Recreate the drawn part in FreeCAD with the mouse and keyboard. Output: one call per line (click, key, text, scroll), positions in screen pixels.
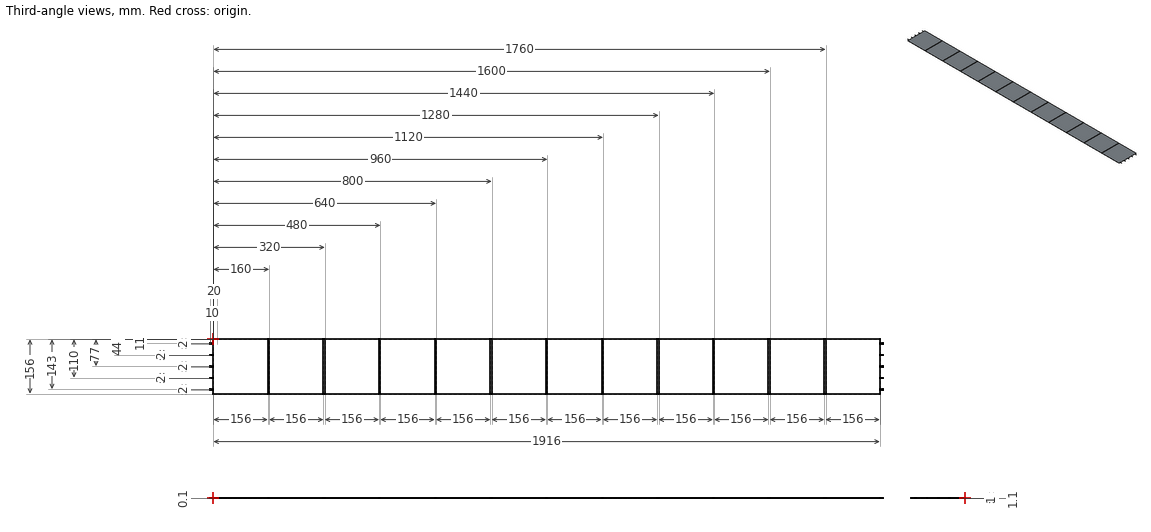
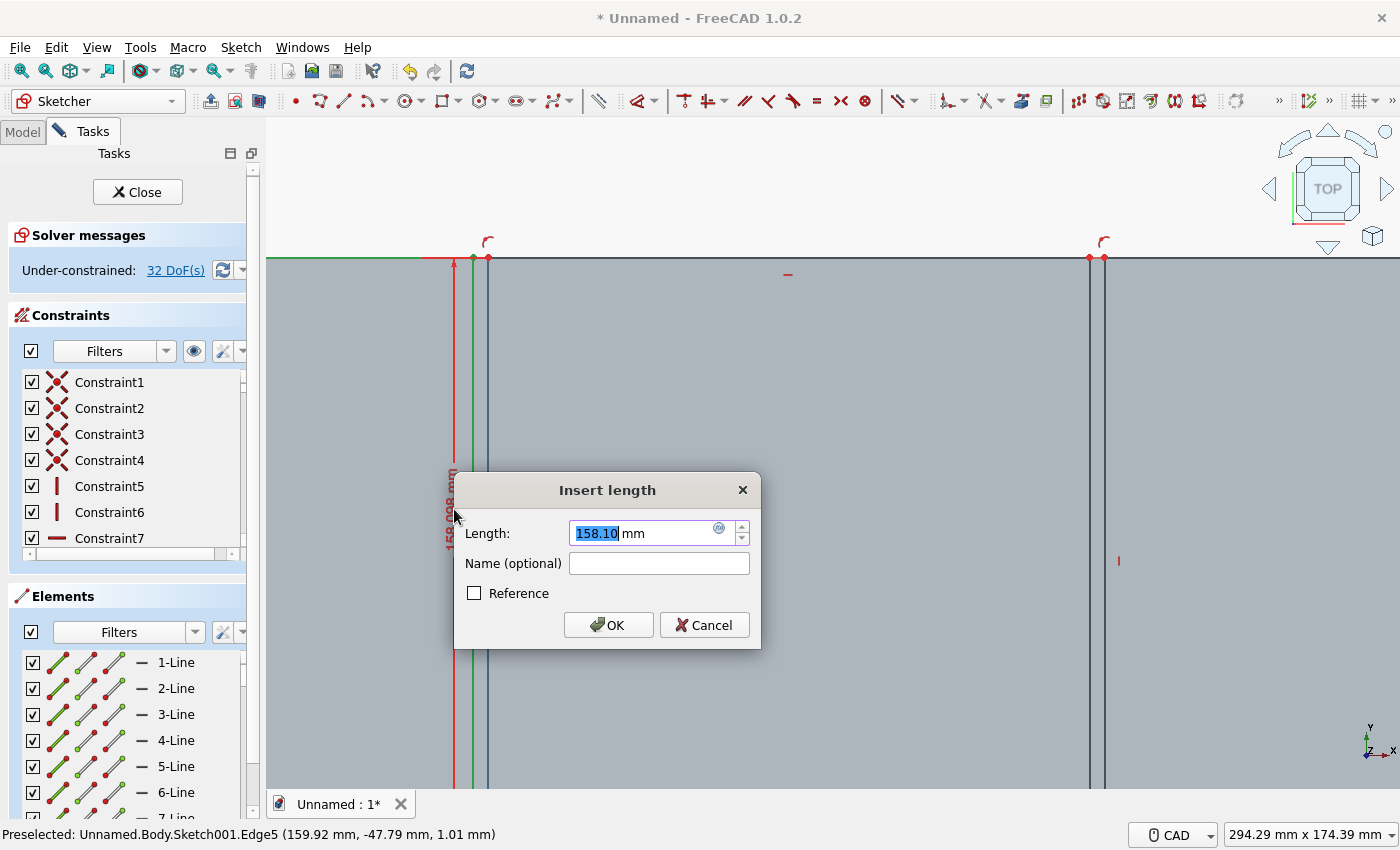
text(156)
key(Return)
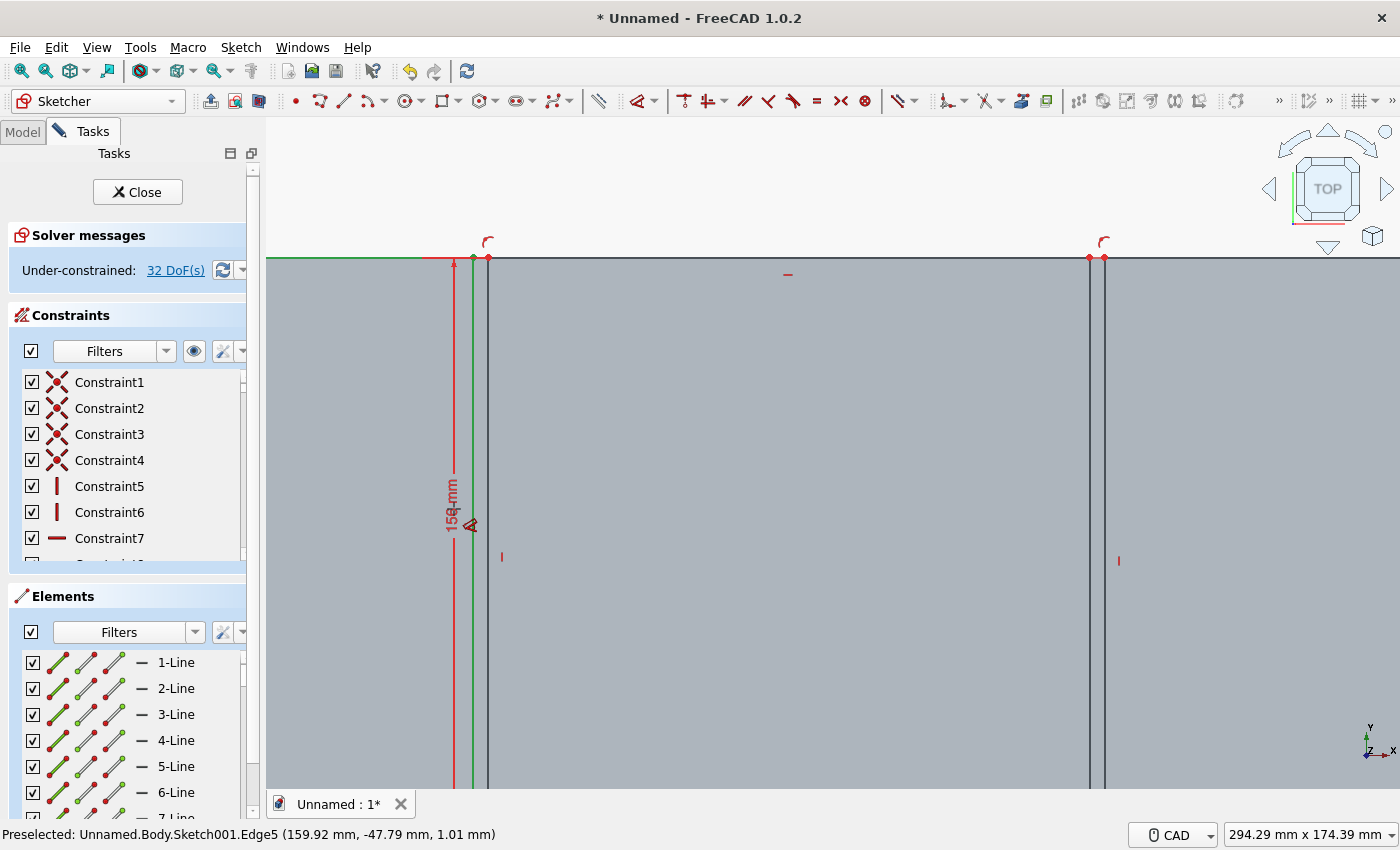
scroll(485, 442, down, 12)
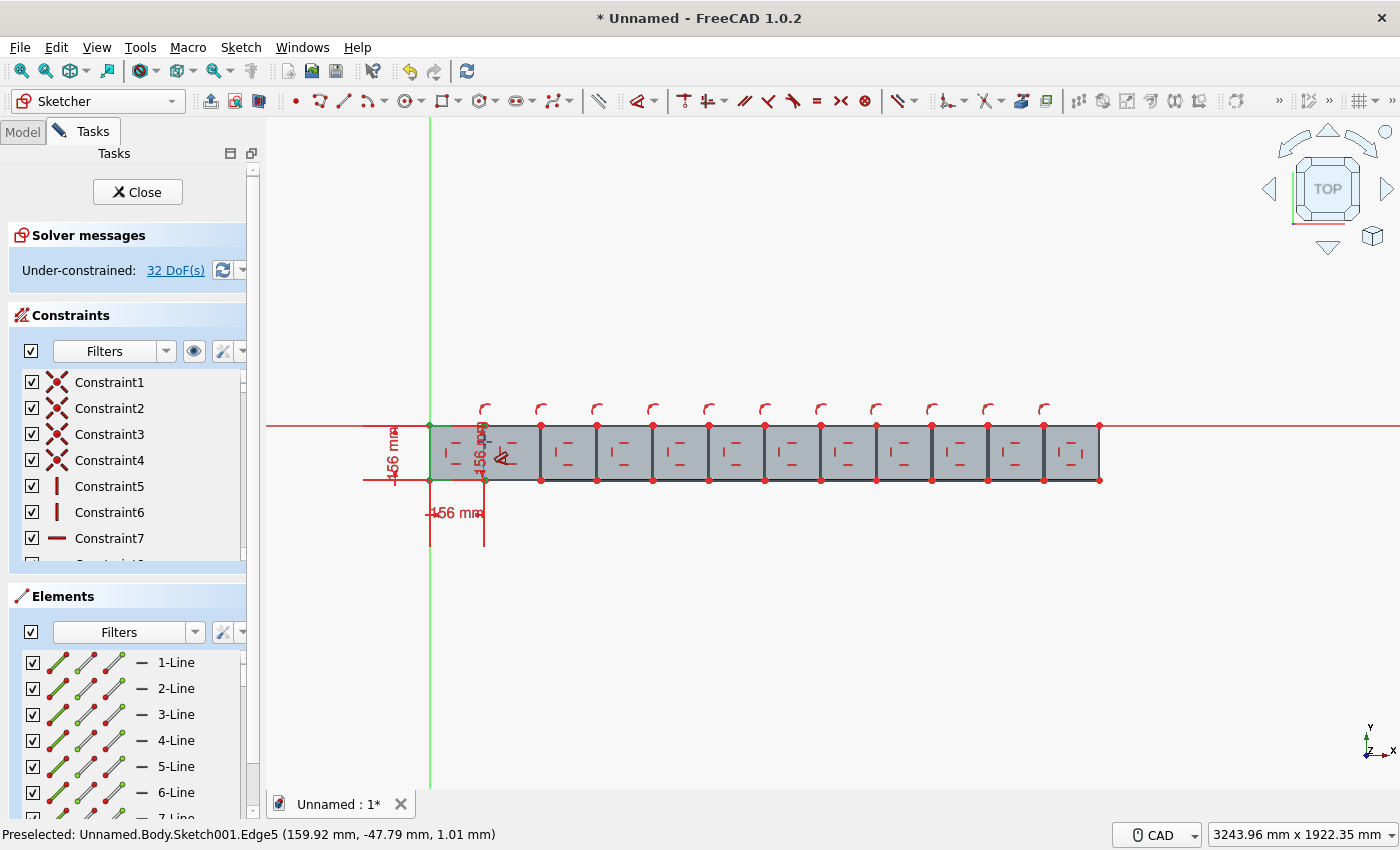
click(502, 480)
click(532, 514)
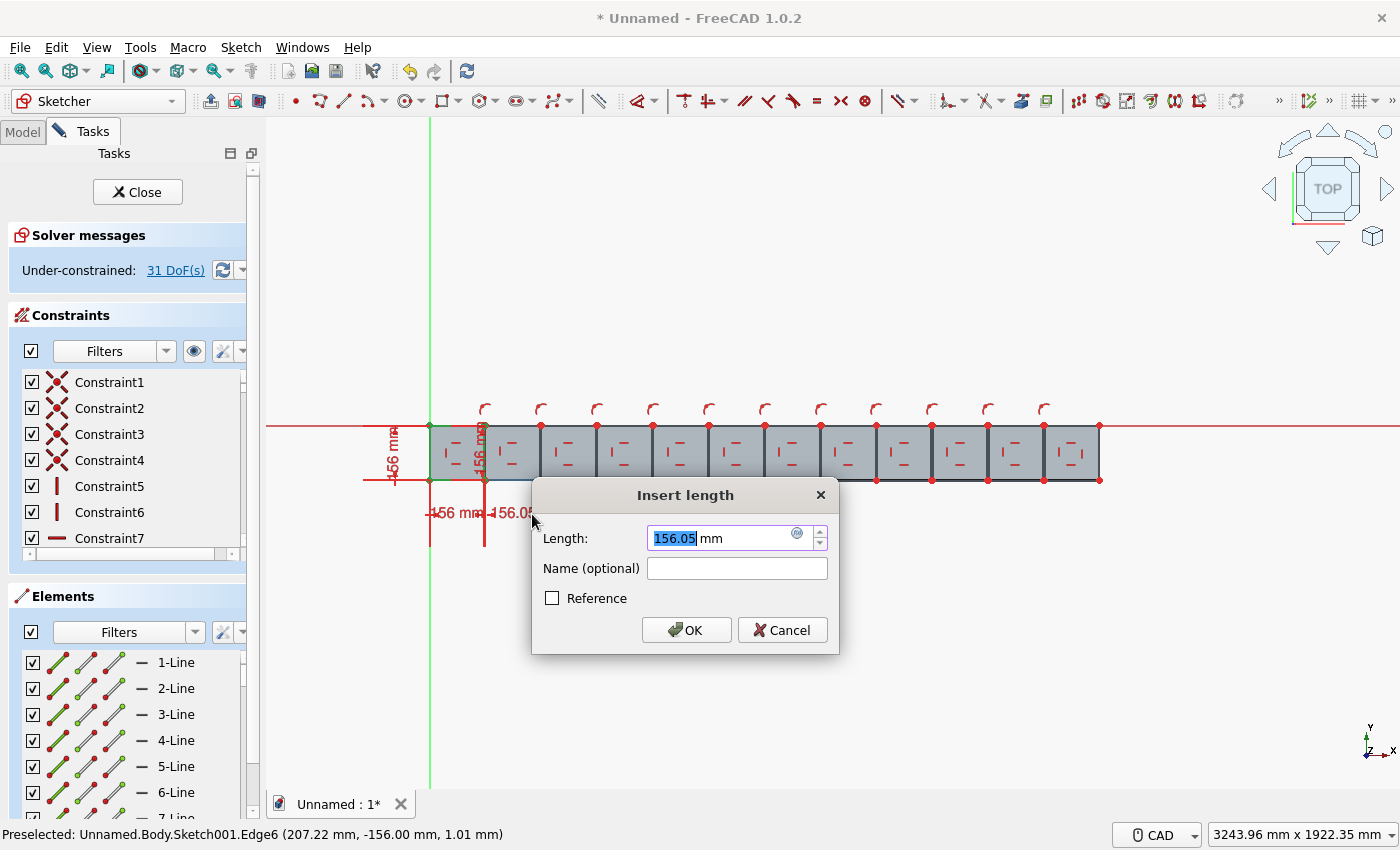
text(156)
key(Return)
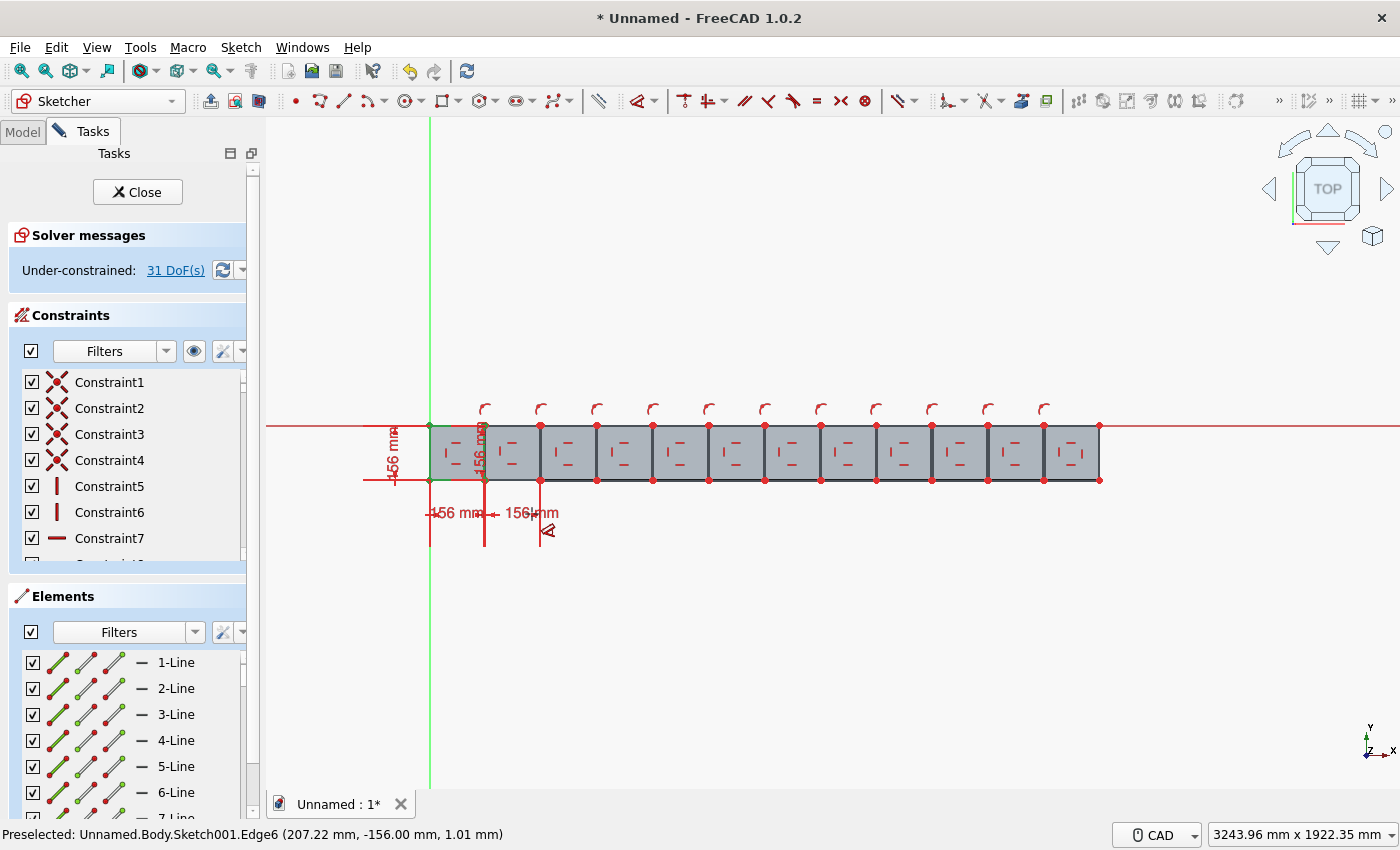
scroll(541, 442, up, 12)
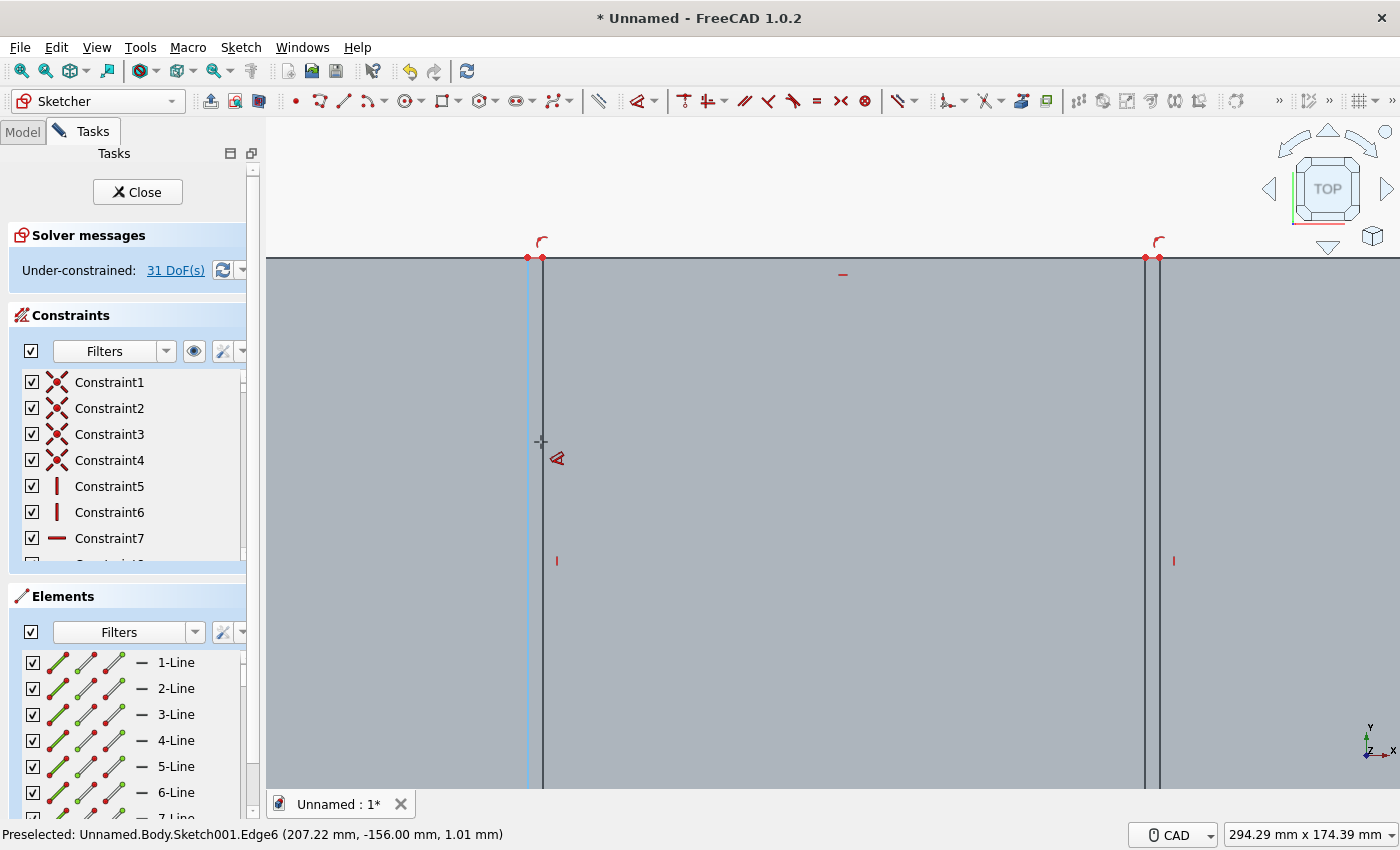
click(543, 441)
click(509, 509)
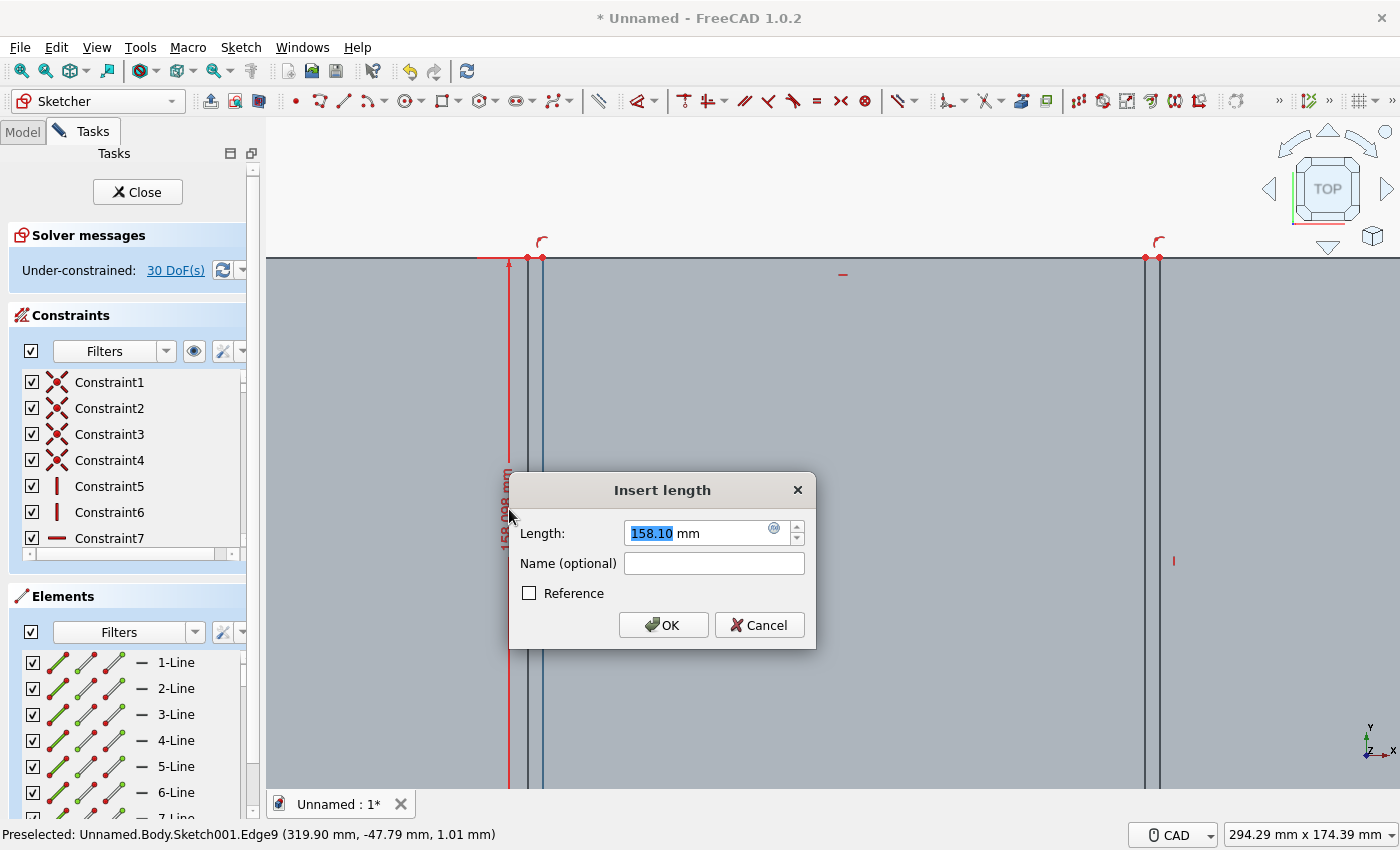
text(156)
key(Return)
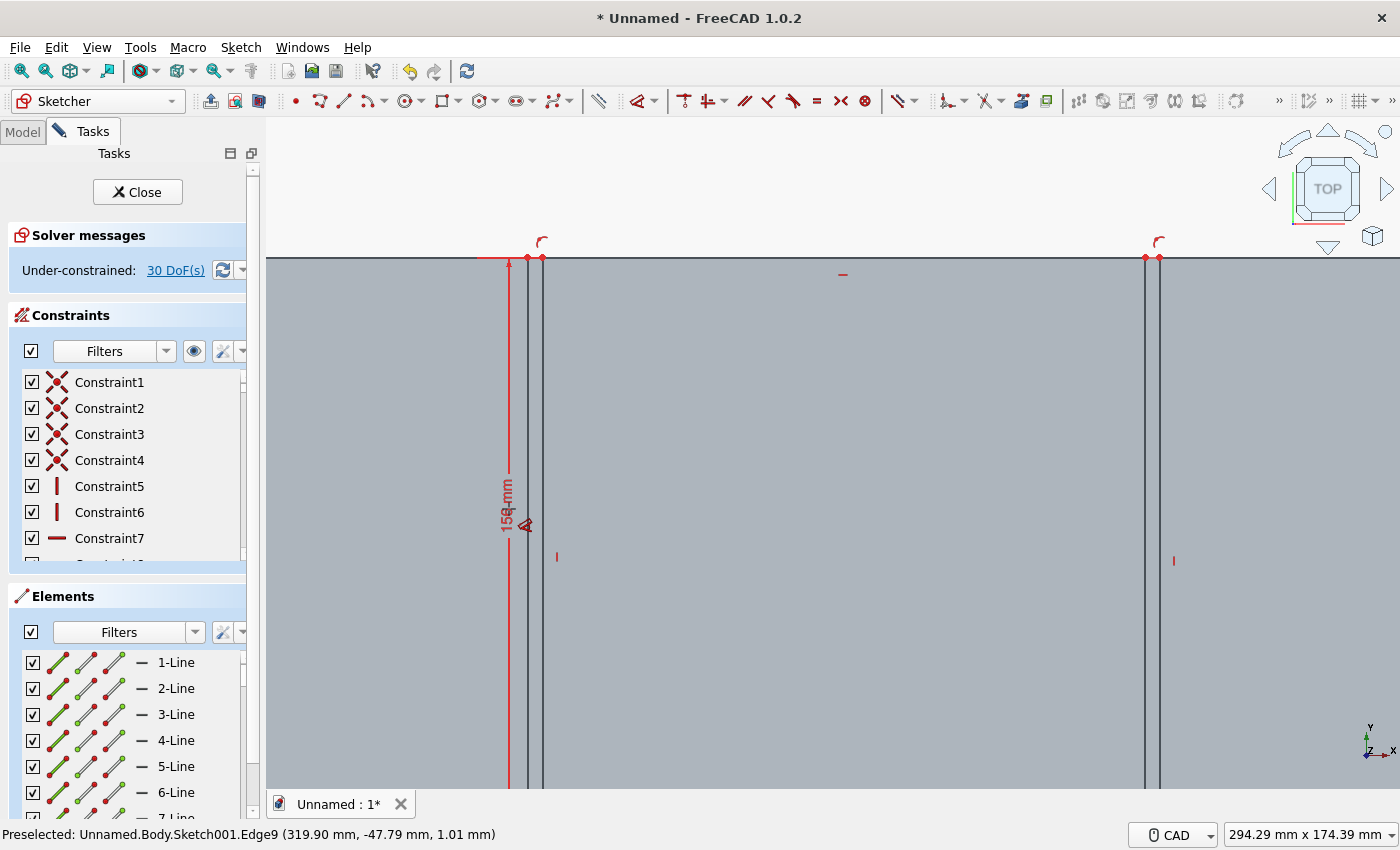
scroll(541, 442, down, 12)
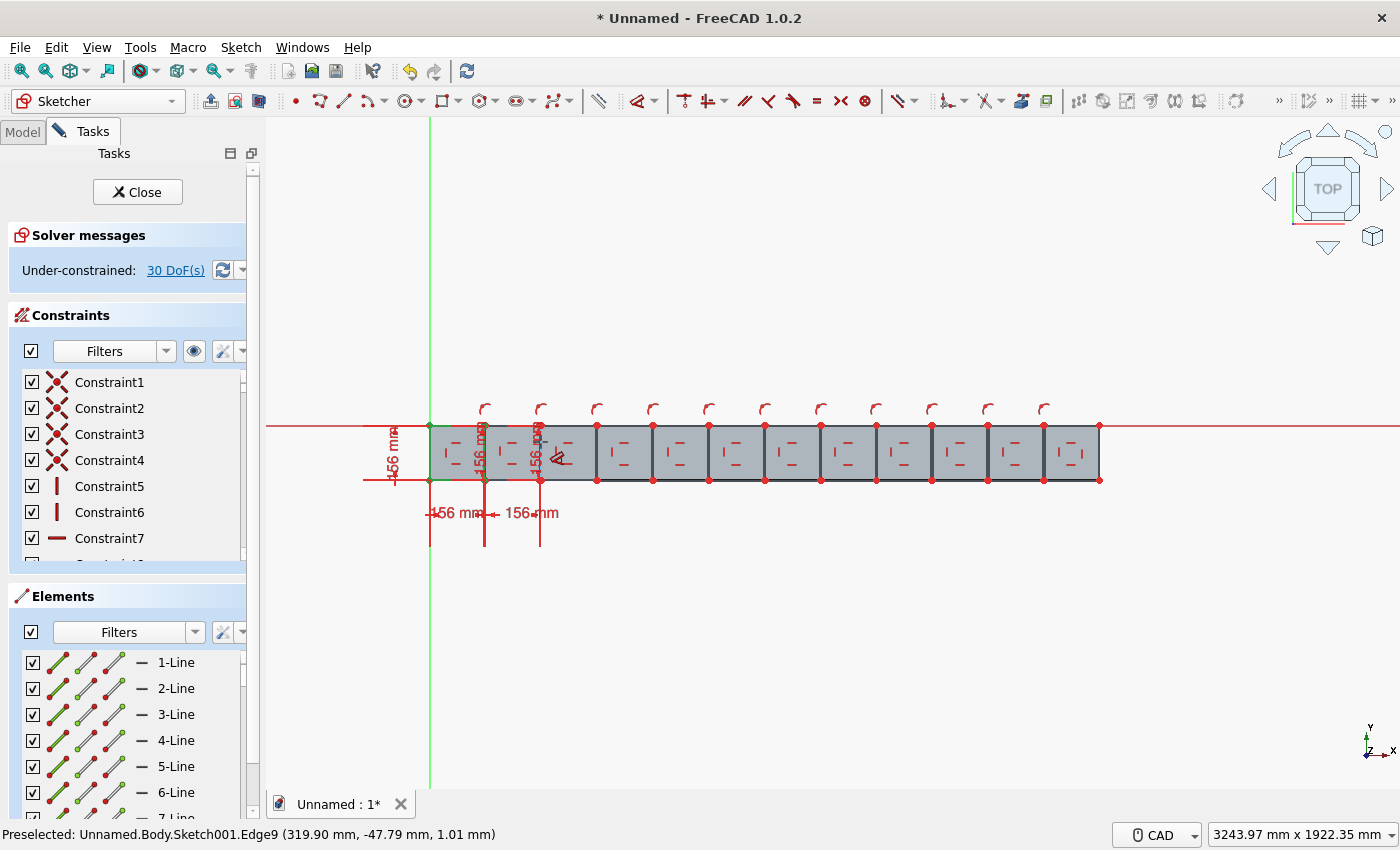
click(558, 480)
click(569, 538)